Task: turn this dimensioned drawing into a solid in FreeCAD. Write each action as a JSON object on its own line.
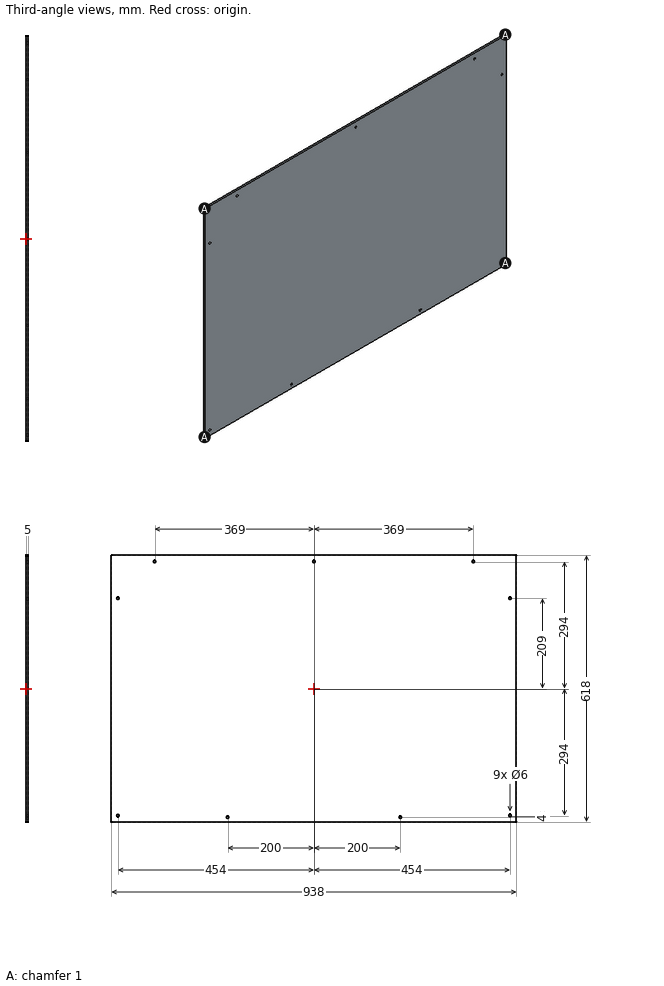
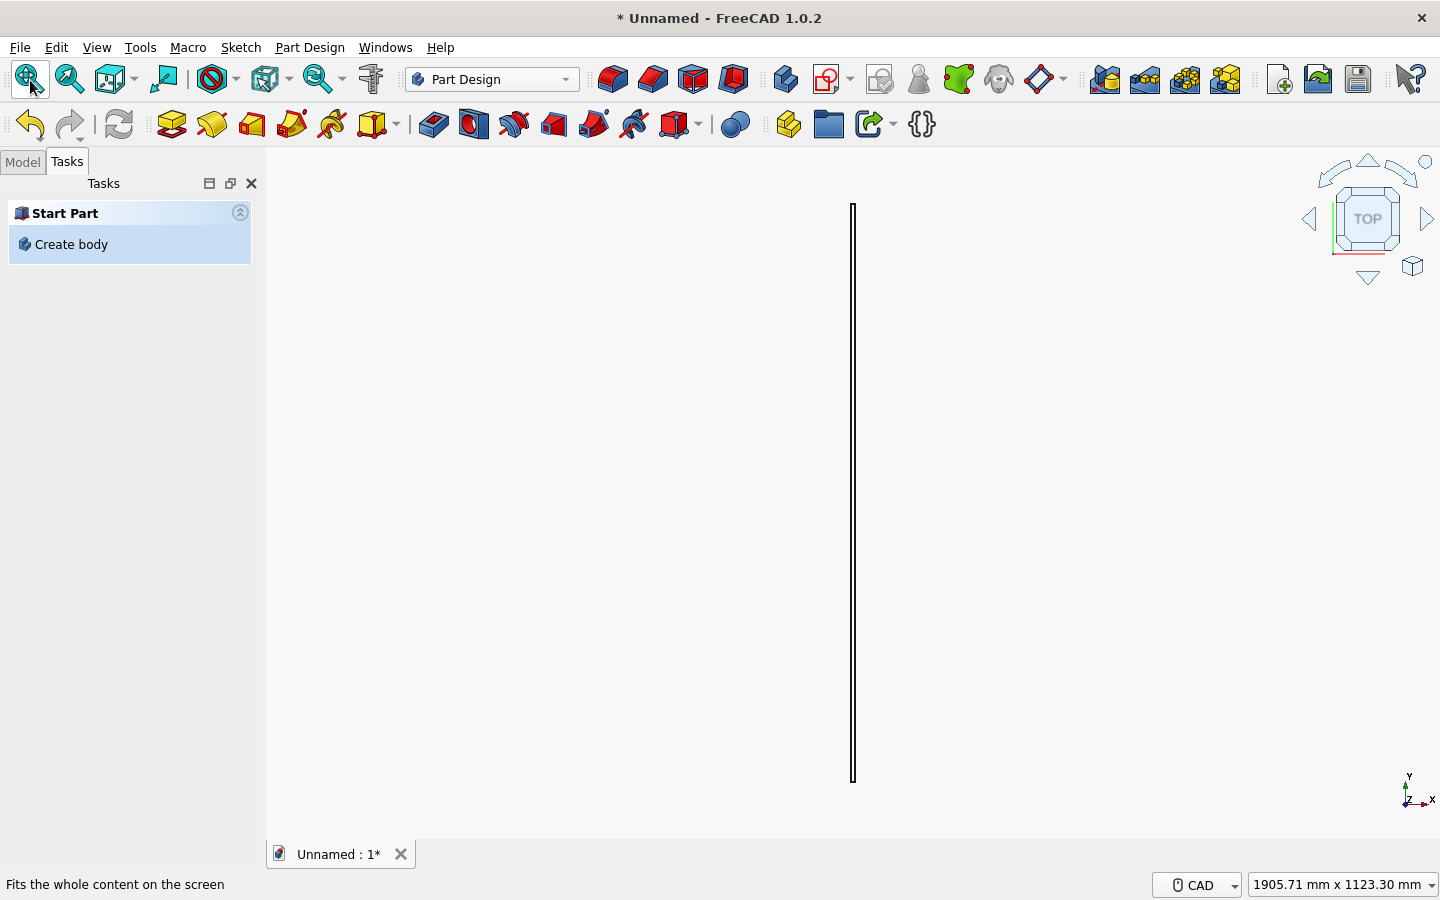
{"action": "scroll", "coordinate": [853, 203], "scroll_direction": "up", "scroll_amount": 13}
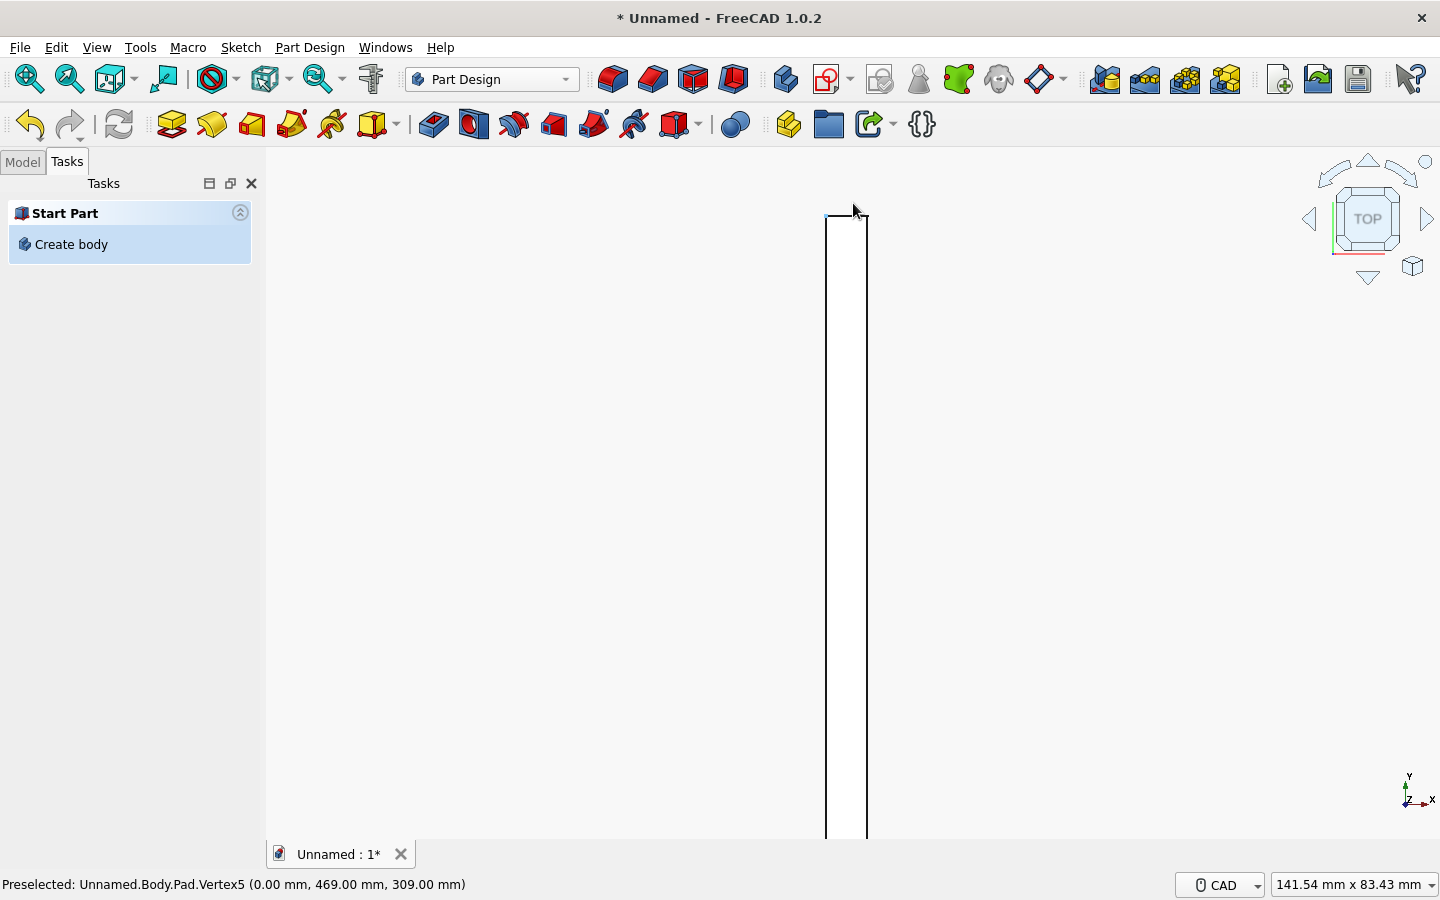
{"action": "left_click", "coordinate": [847, 215]}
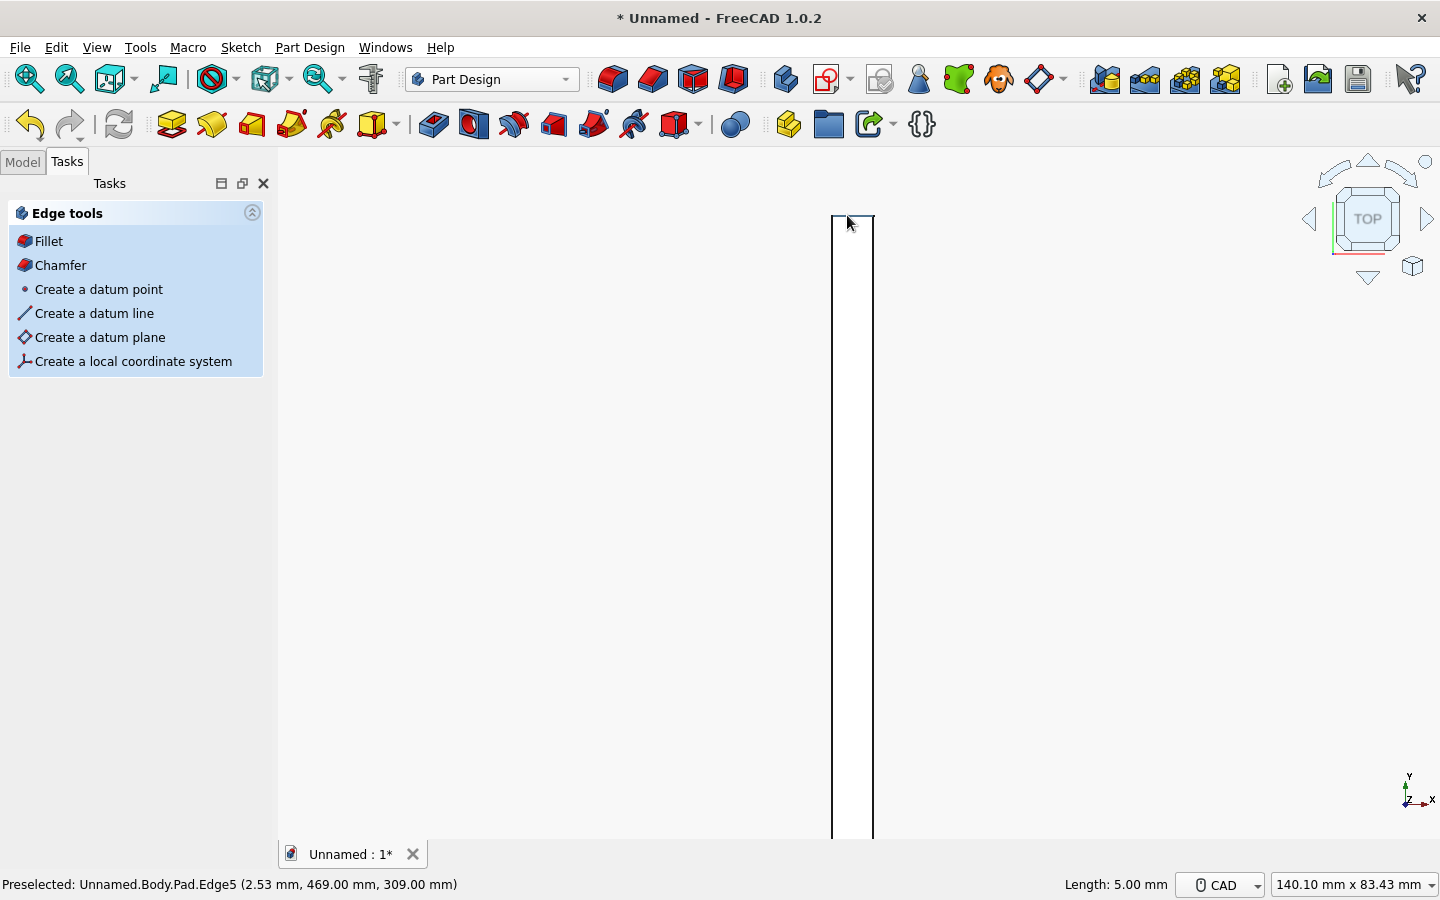
{"action": "left_click", "coordinate": [30, 80]}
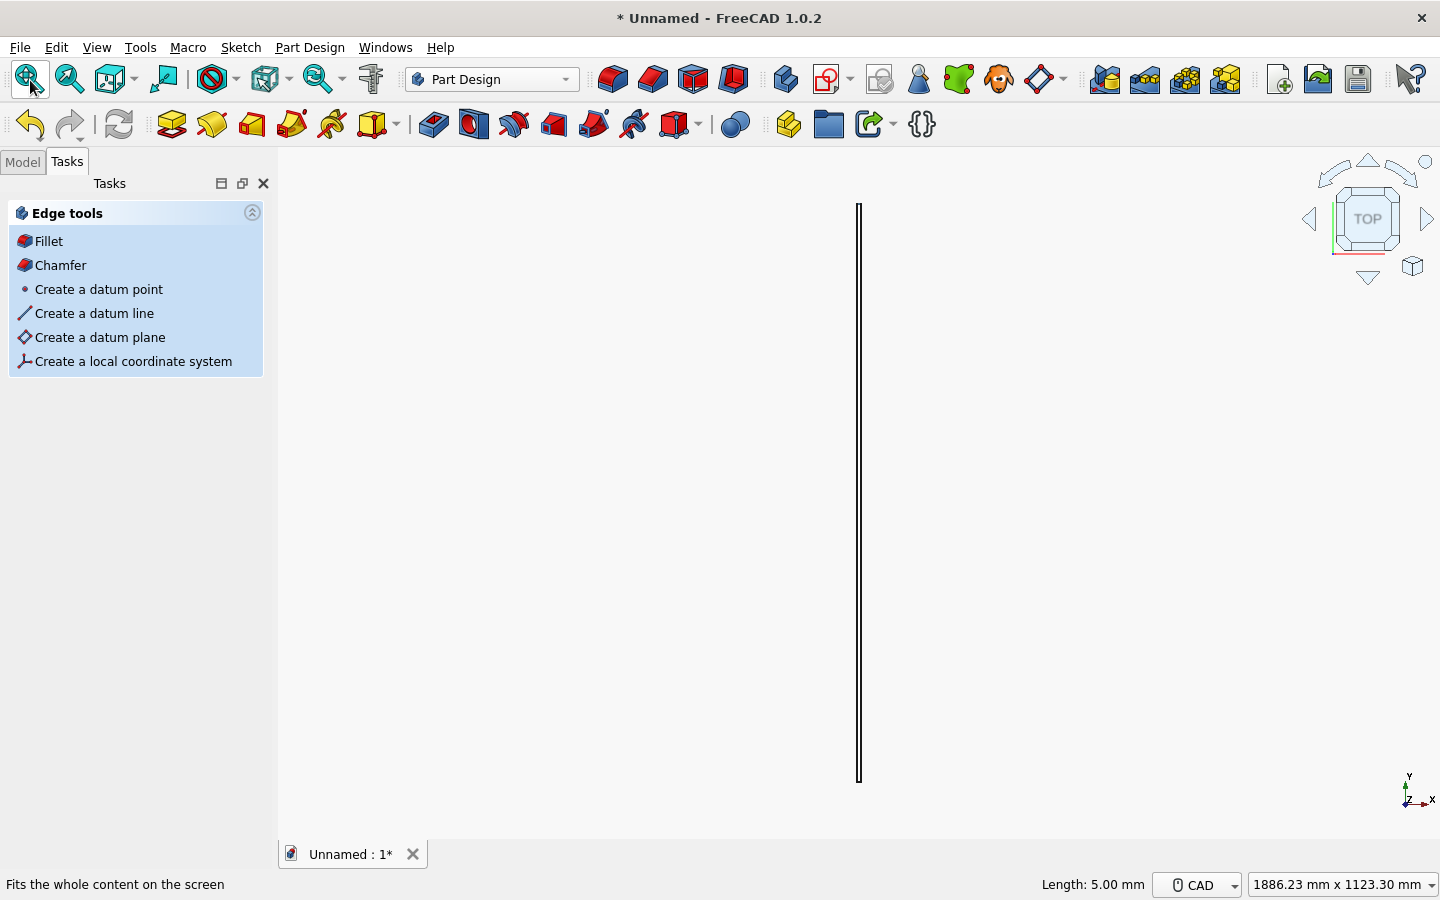
{"action": "key", "text": "1"}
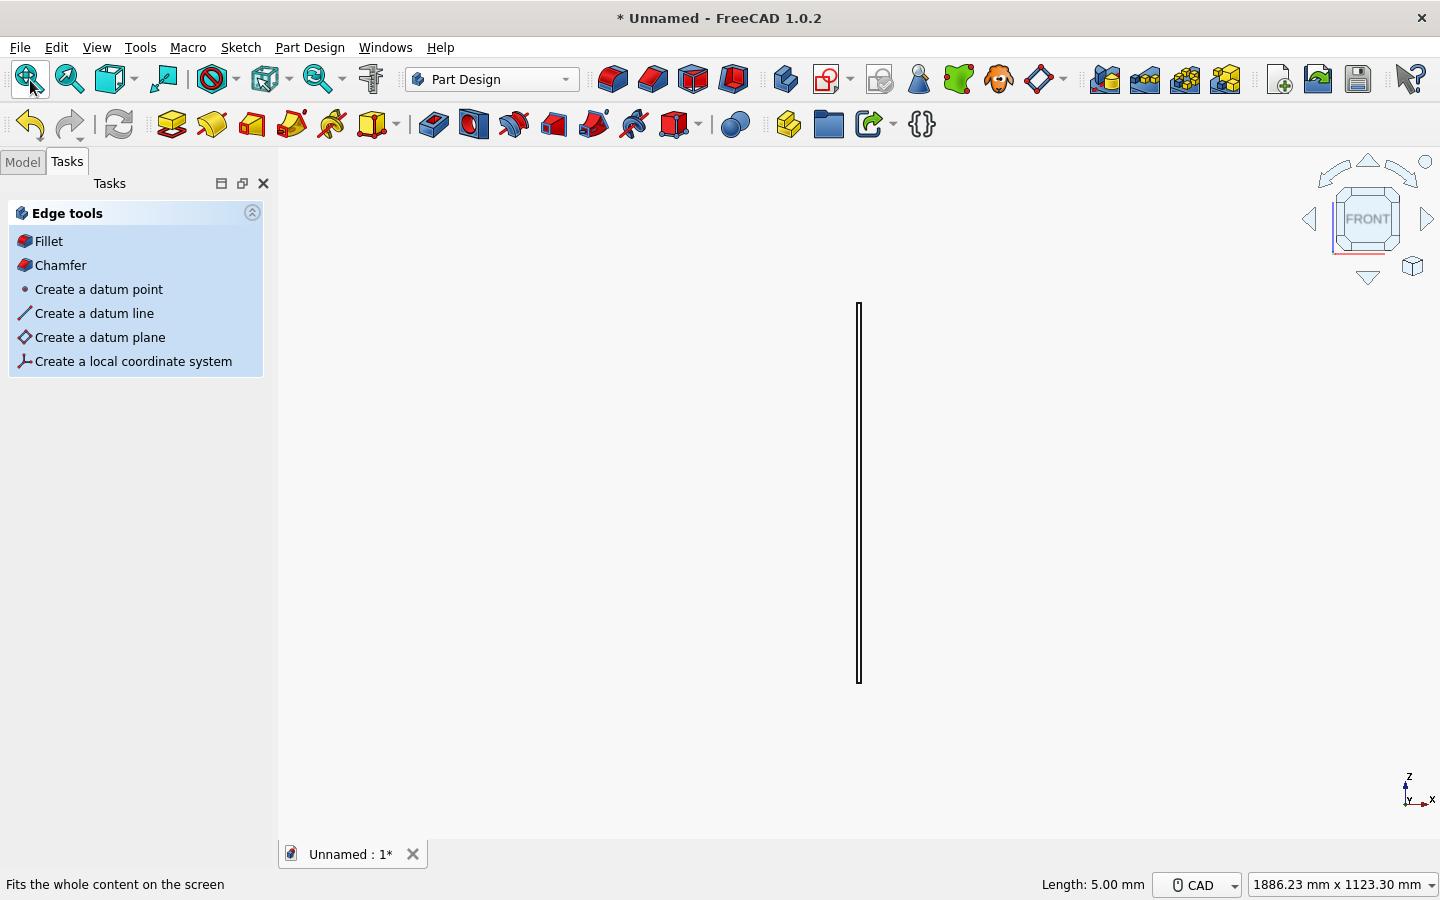
{"action": "scroll", "coordinate": [859, 682], "scroll_direction": "up", "scroll_amount": 13}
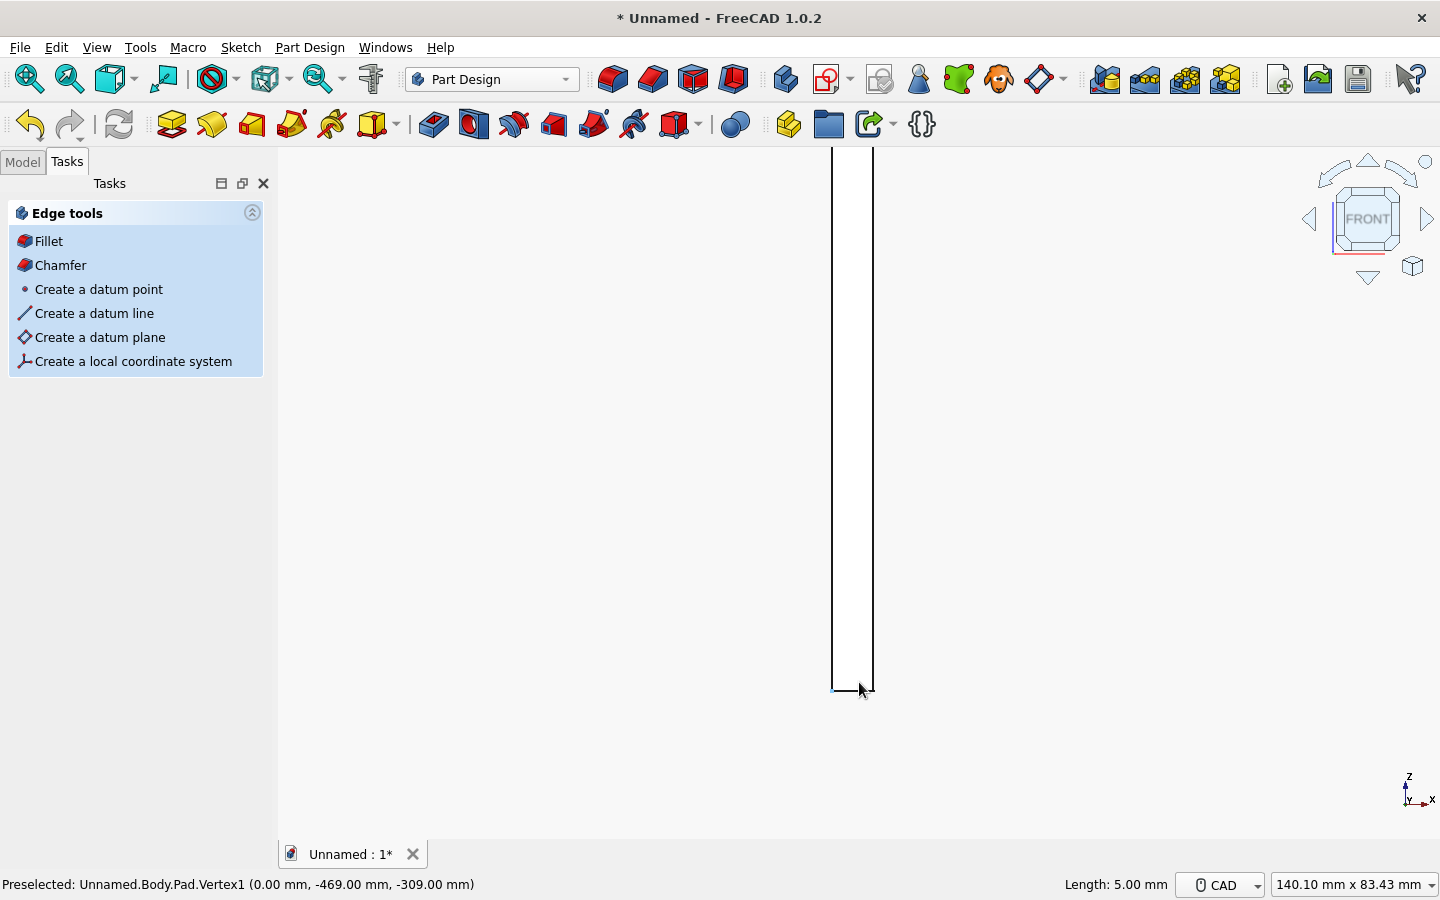
{"action": "left_click", "coordinate": [853, 690], "text": "ctrl"}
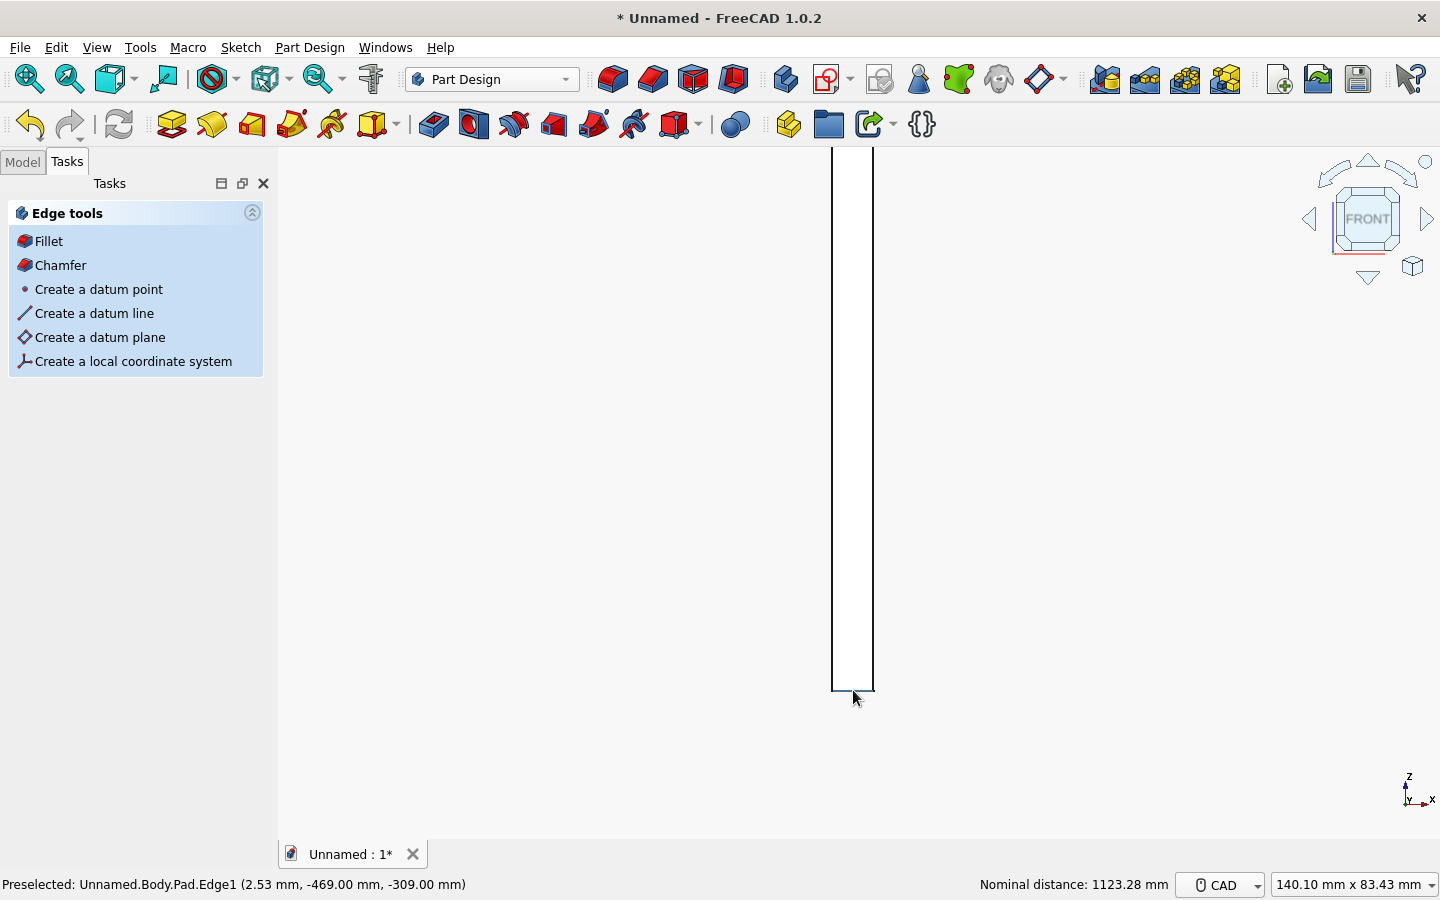
{"action": "left_click", "coordinate": [30, 80]}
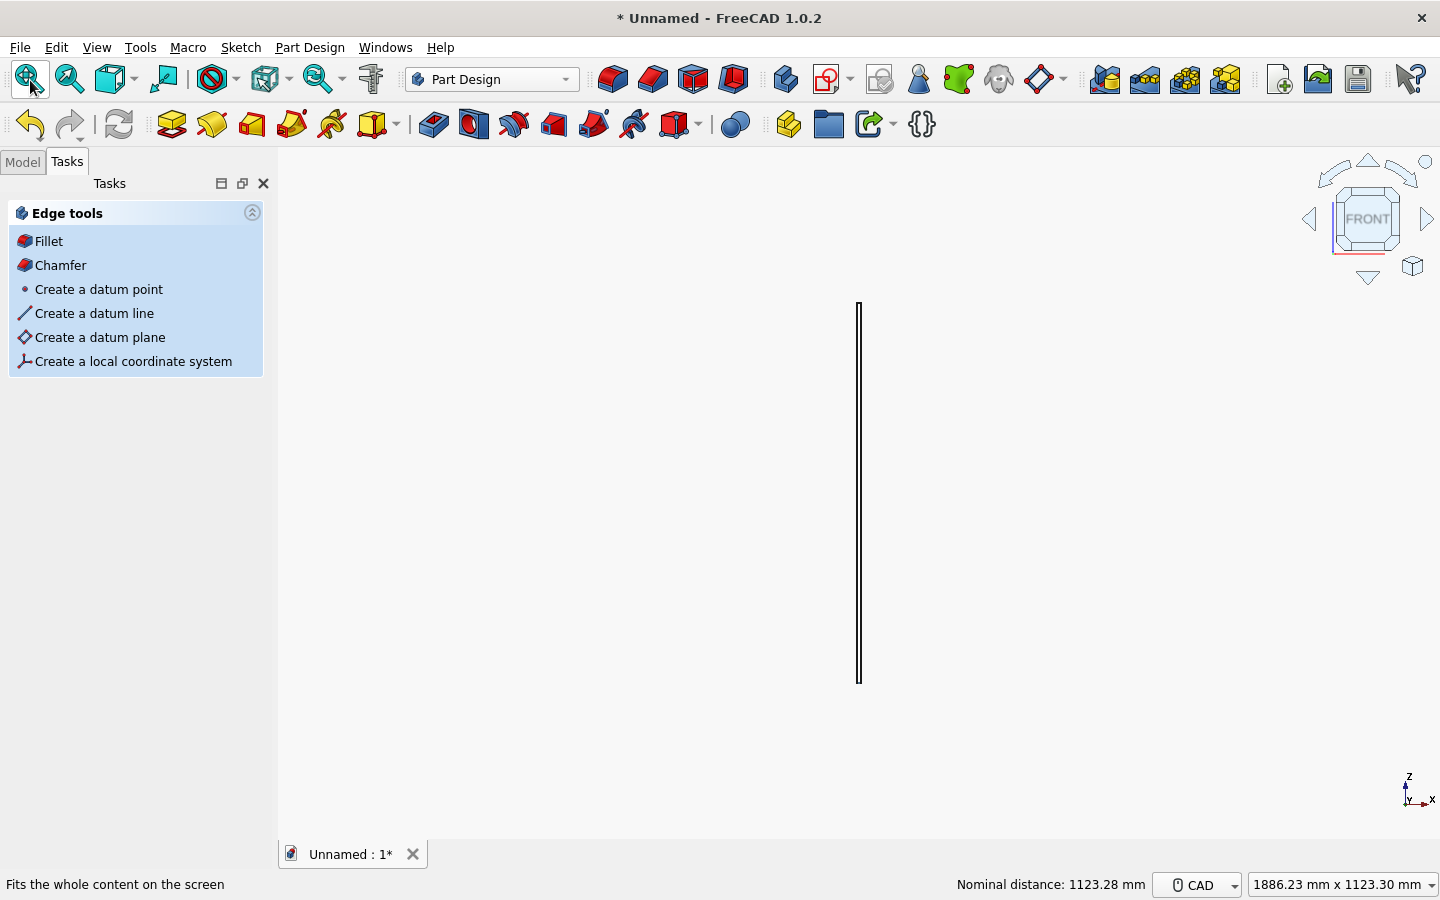
{"action": "key", "text": "3"}